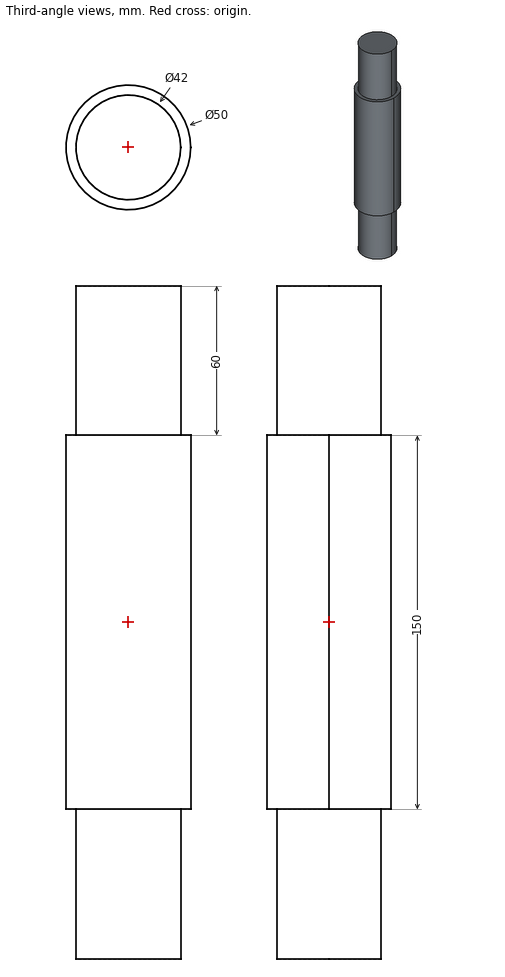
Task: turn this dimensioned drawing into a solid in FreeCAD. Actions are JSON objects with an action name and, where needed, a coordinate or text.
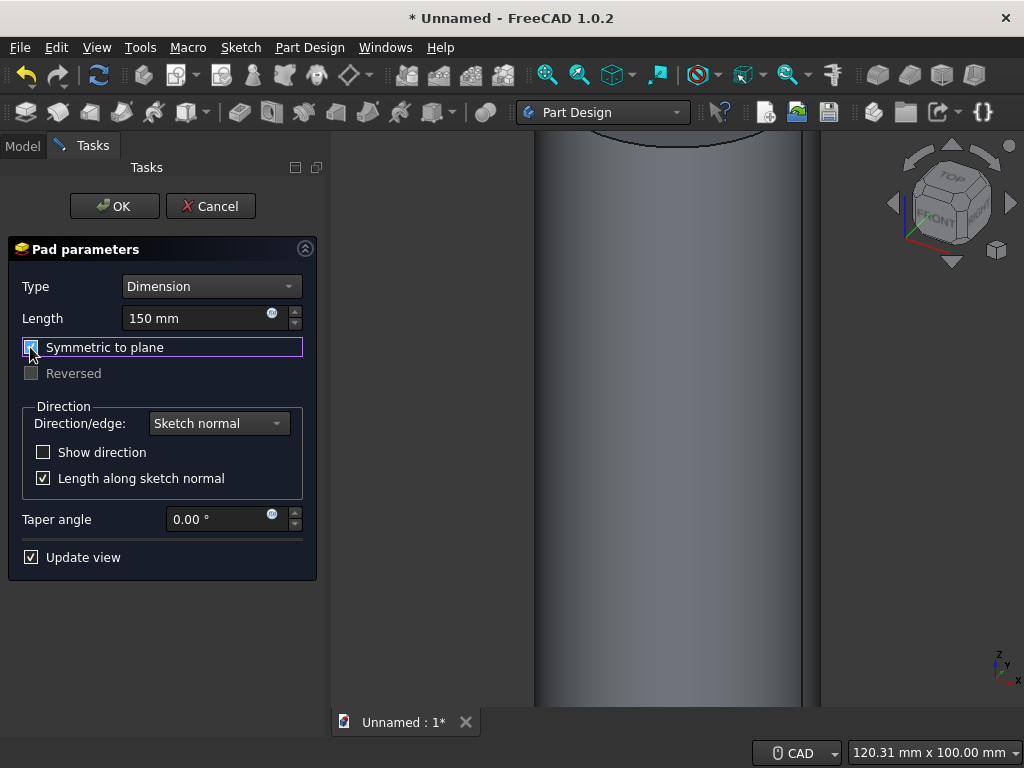
{"action": "left_click", "coordinate": [115, 206]}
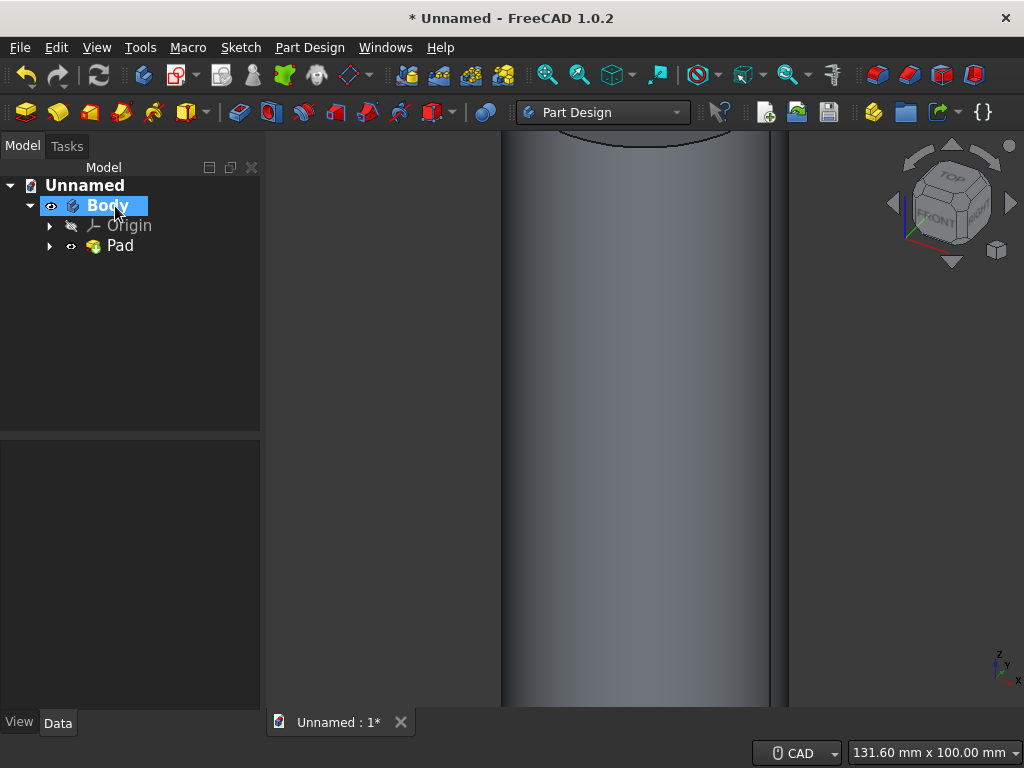
{"action": "left_click", "coordinate": [548, 76]}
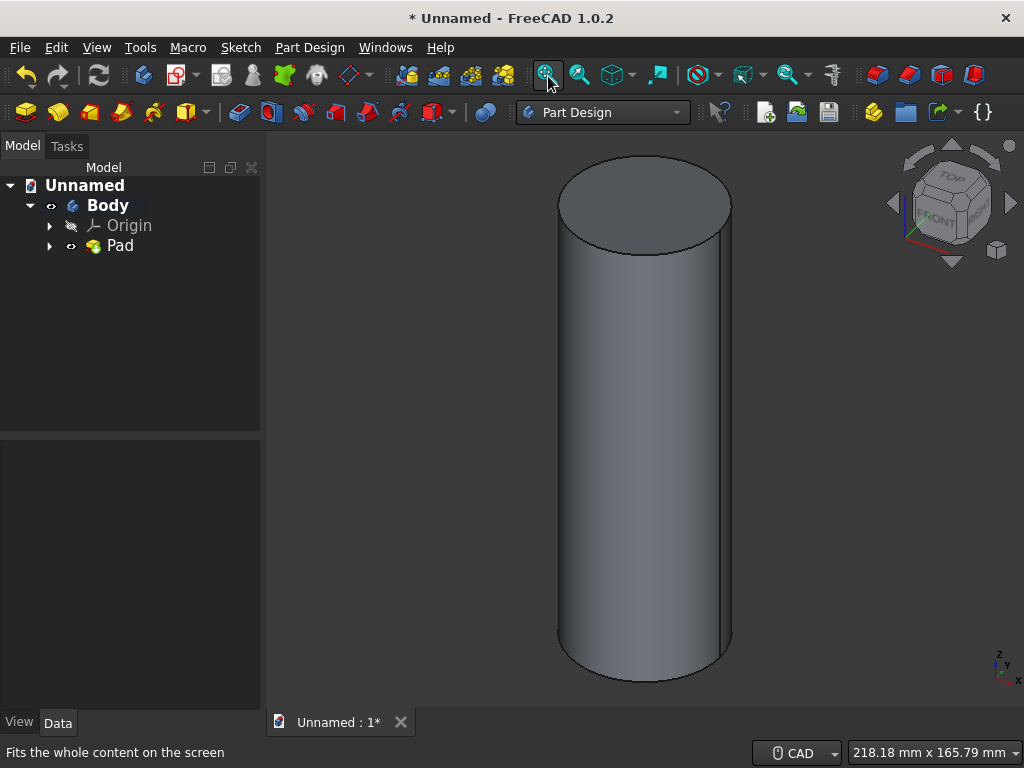
{"action": "left_click", "coordinate": [645, 205]}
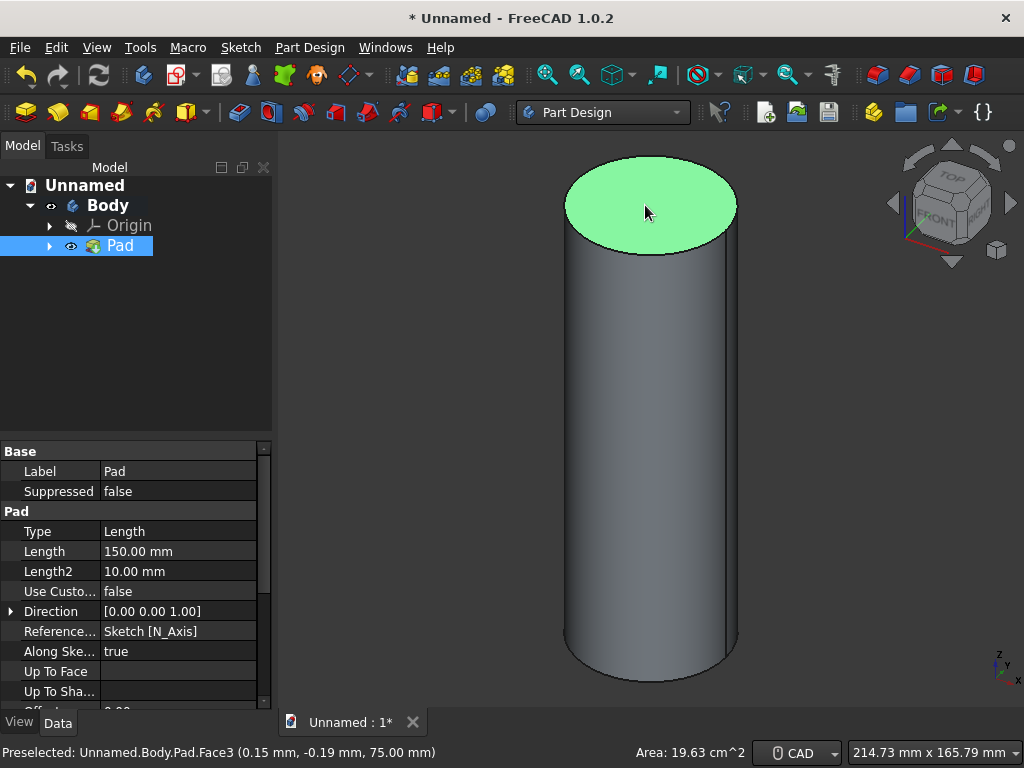
{"action": "left_click", "coordinate": [176, 76]}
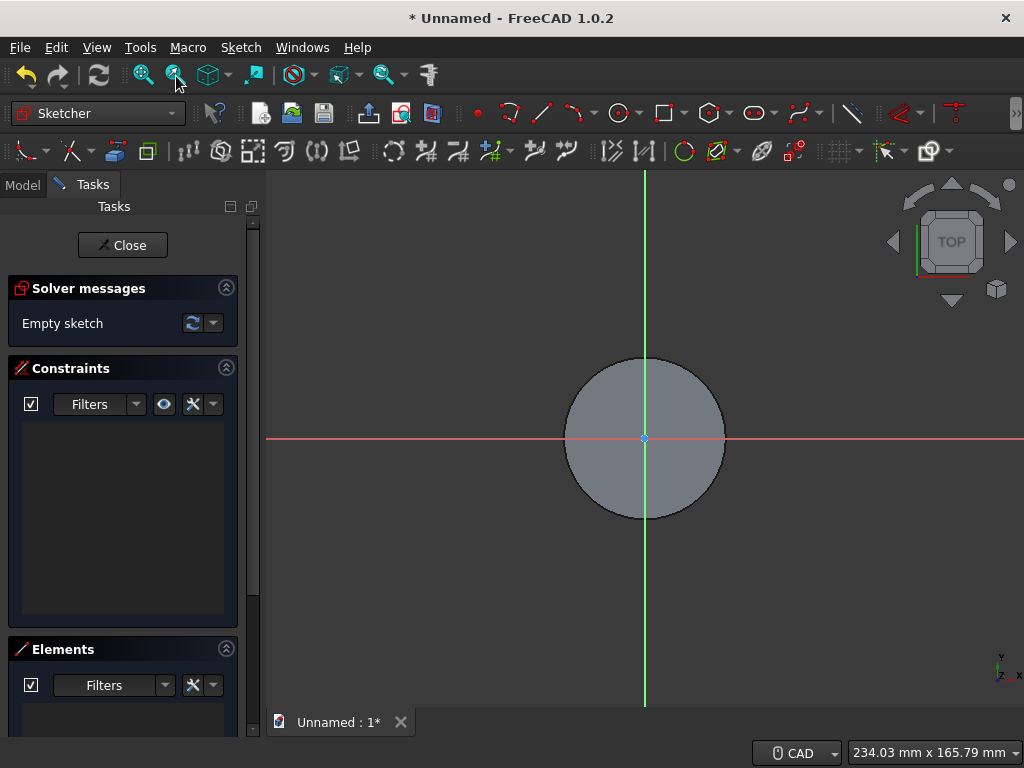
{"action": "scroll", "coordinate": [685, 439], "scroll_direction": "up", "scroll_amount": 5}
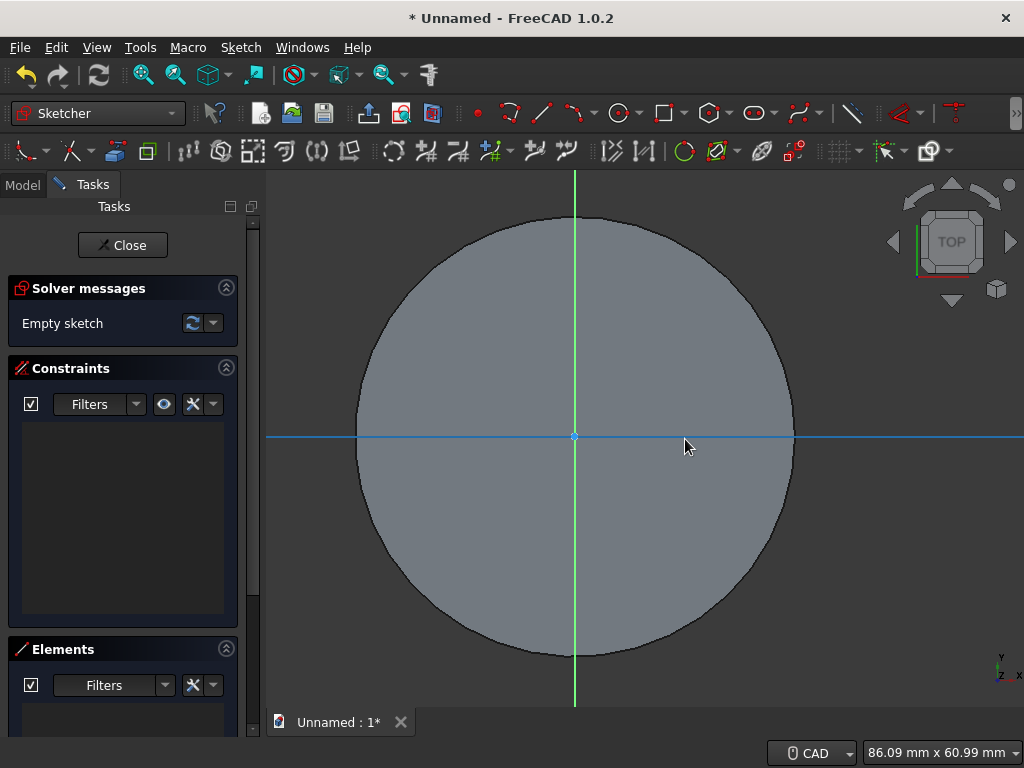
{"action": "left_click", "coordinate": [620, 114]}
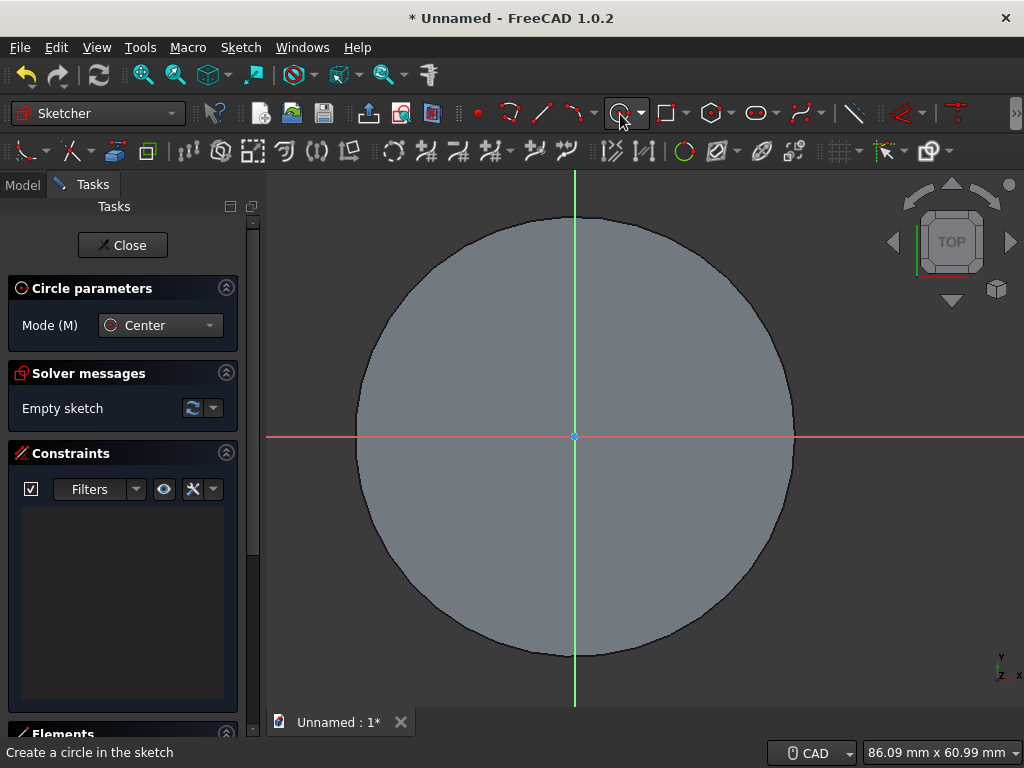
{"action": "left_click", "coordinate": [575, 437]}
{"action": "left_click", "coordinate": [706, 306]}
{"action": "key", "text": "Escape"}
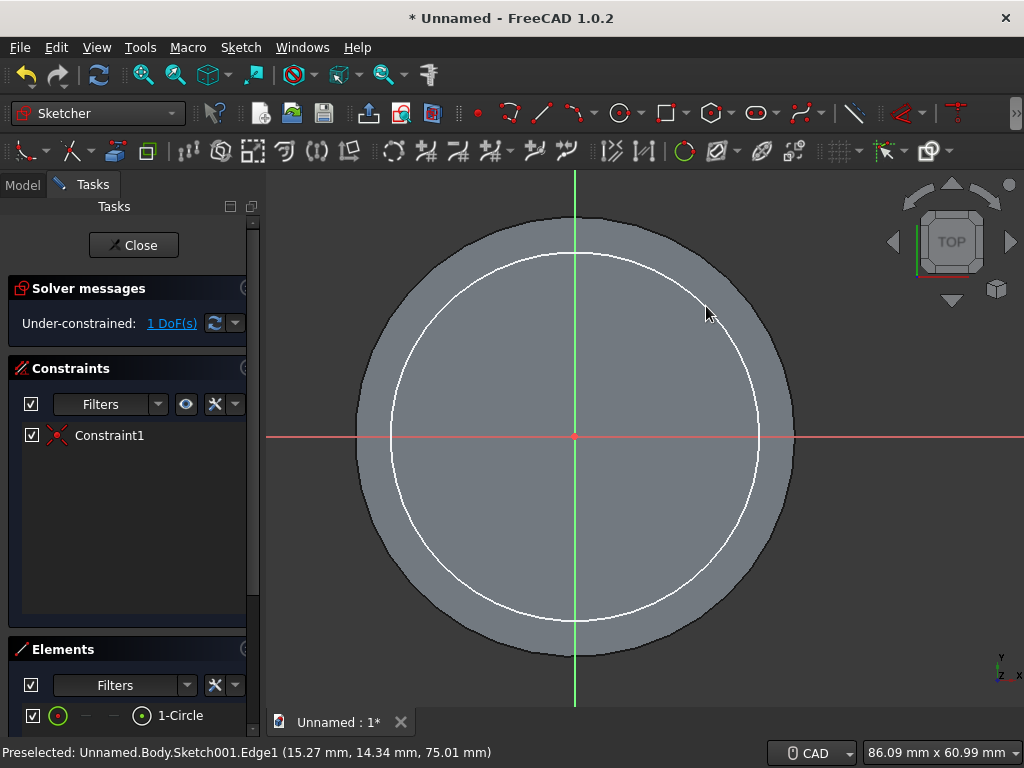
{"action": "left_click", "coordinate": [705, 306]}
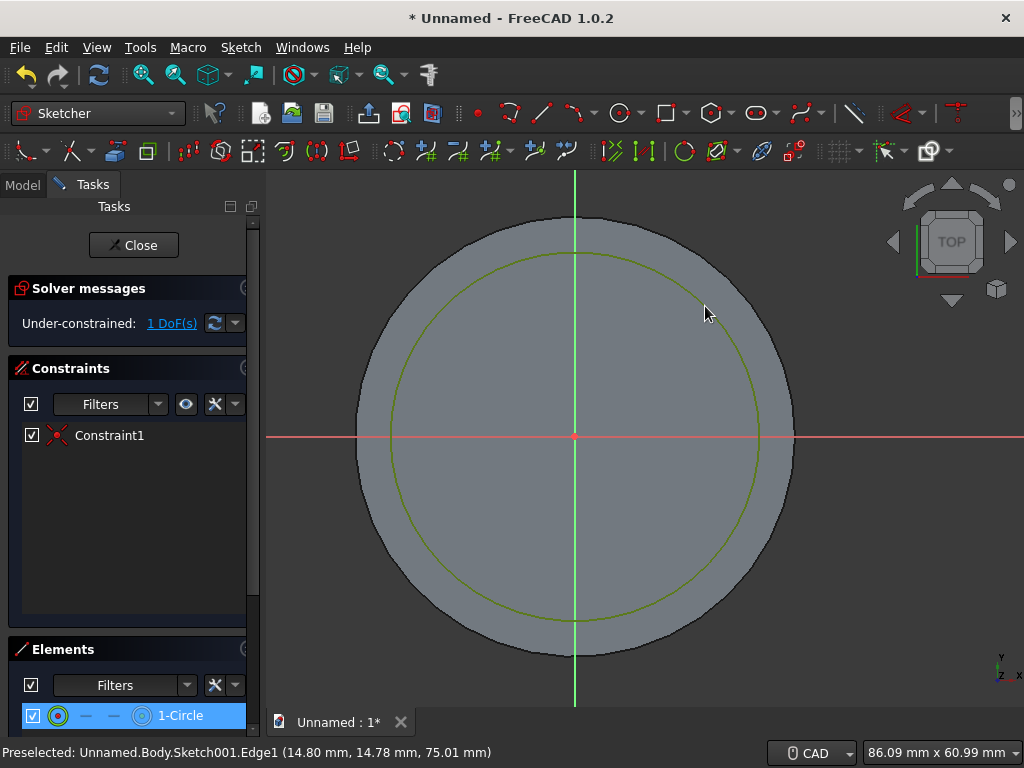
{"action": "left_click", "coordinate": [924, 114]}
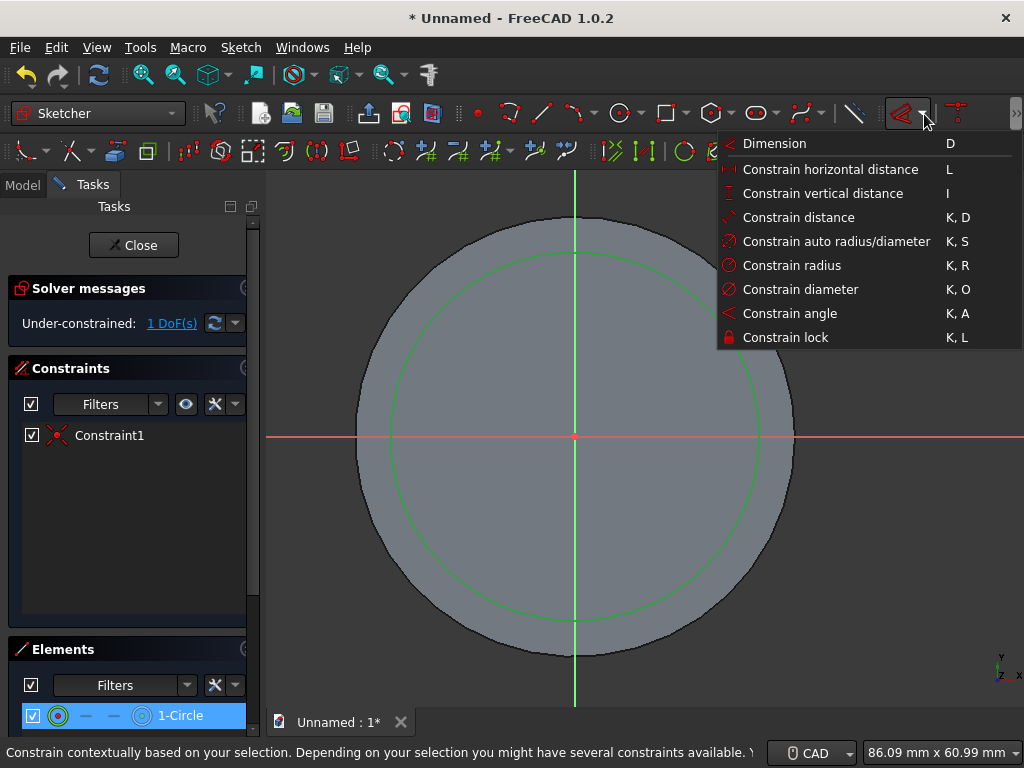
{"action": "left_click", "coordinate": [870, 289]}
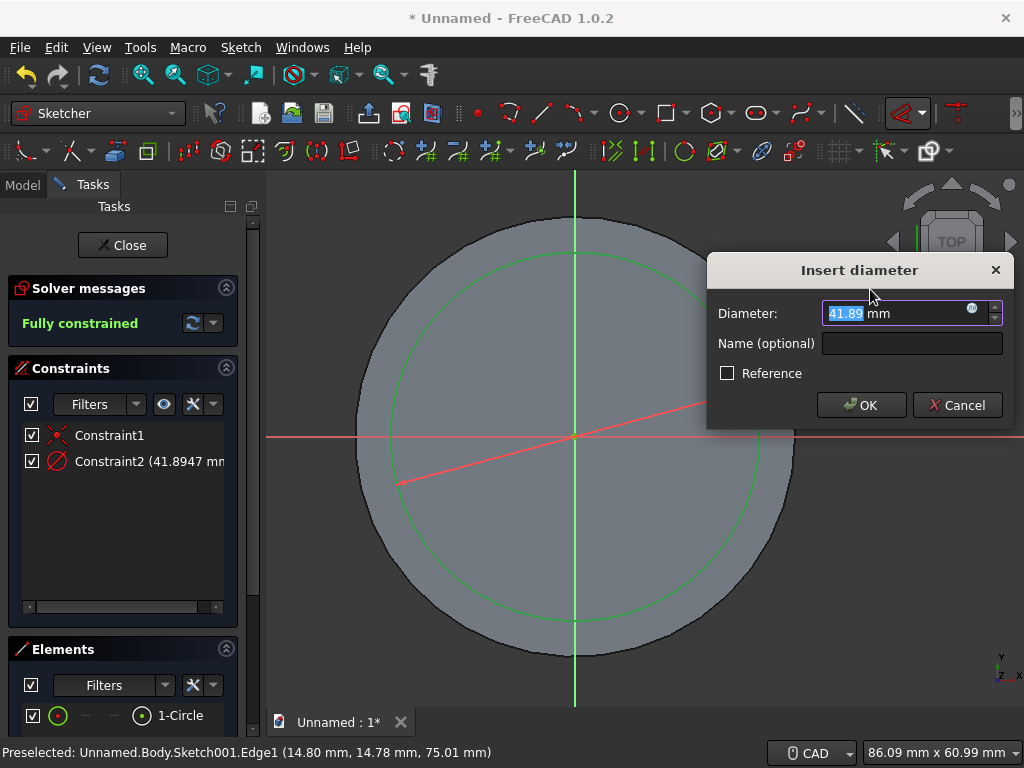
{"action": "type", "text": "42"}
{"action": "key", "text": "Return"}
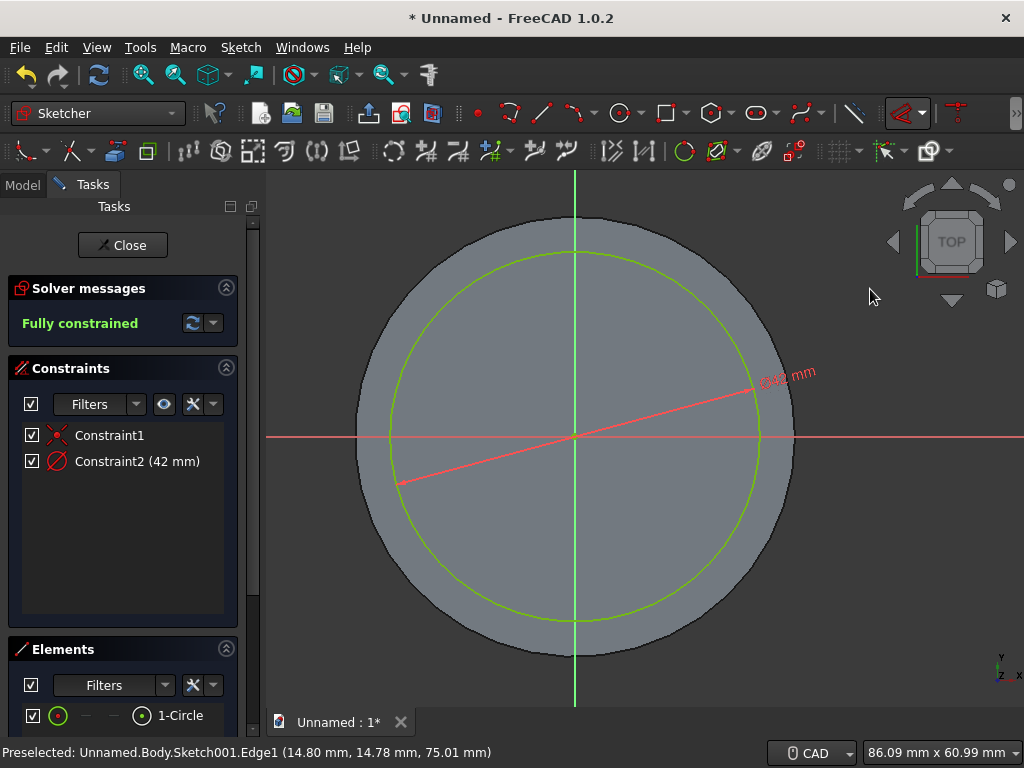
{"action": "left_click", "coordinate": [123, 245]}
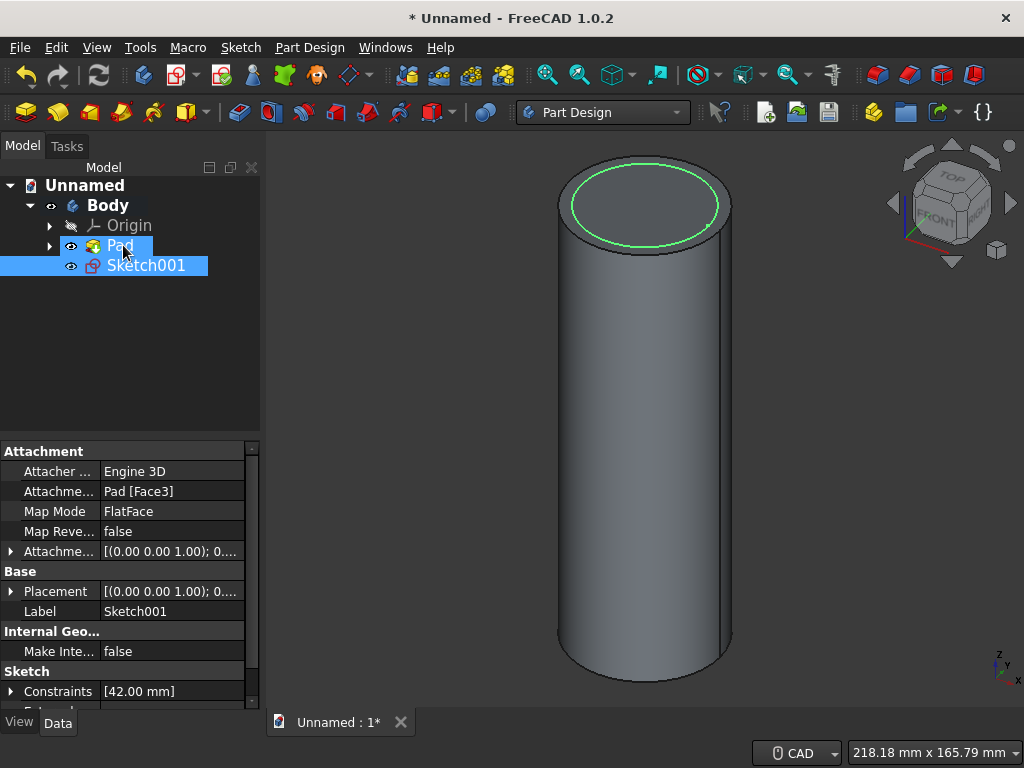
{"action": "left_click", "coordinate": [26, 112]}